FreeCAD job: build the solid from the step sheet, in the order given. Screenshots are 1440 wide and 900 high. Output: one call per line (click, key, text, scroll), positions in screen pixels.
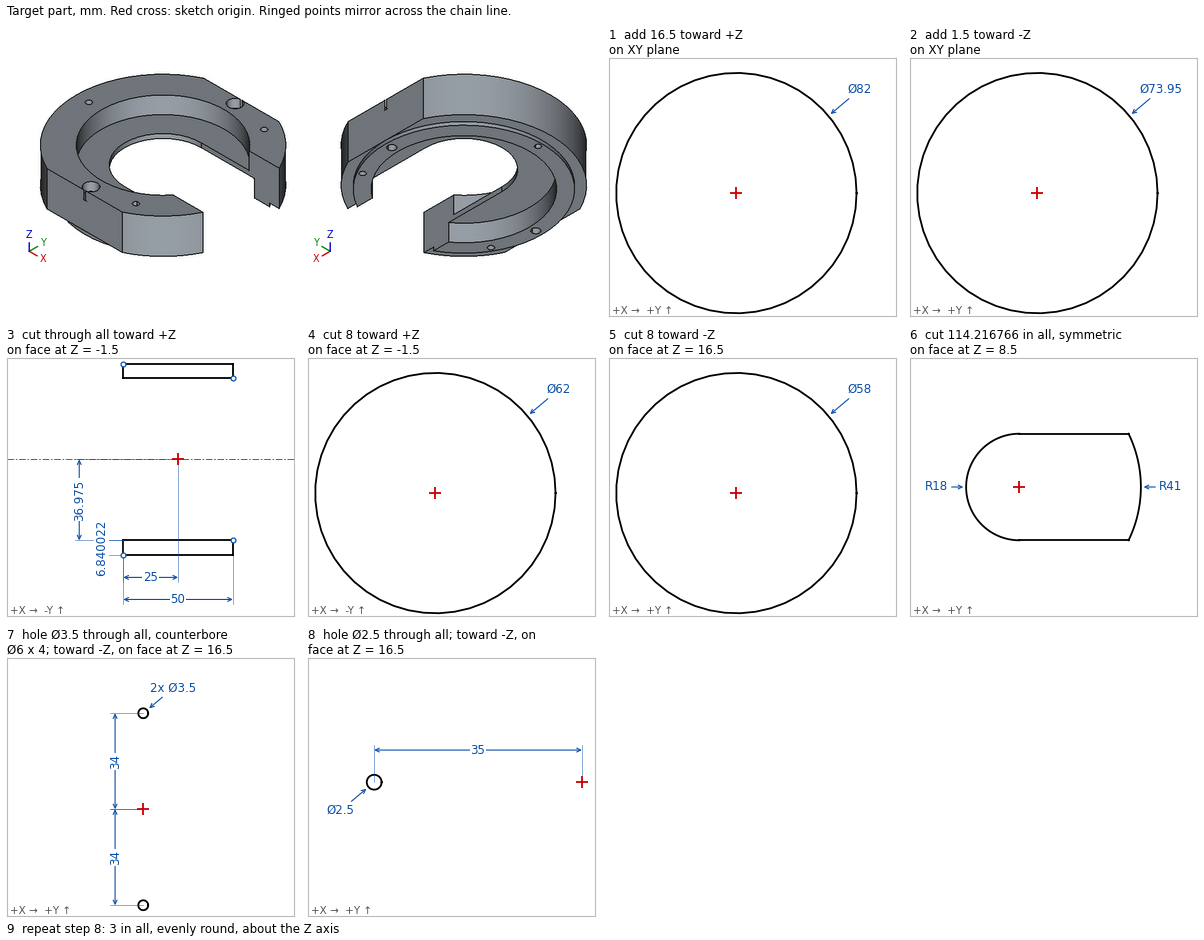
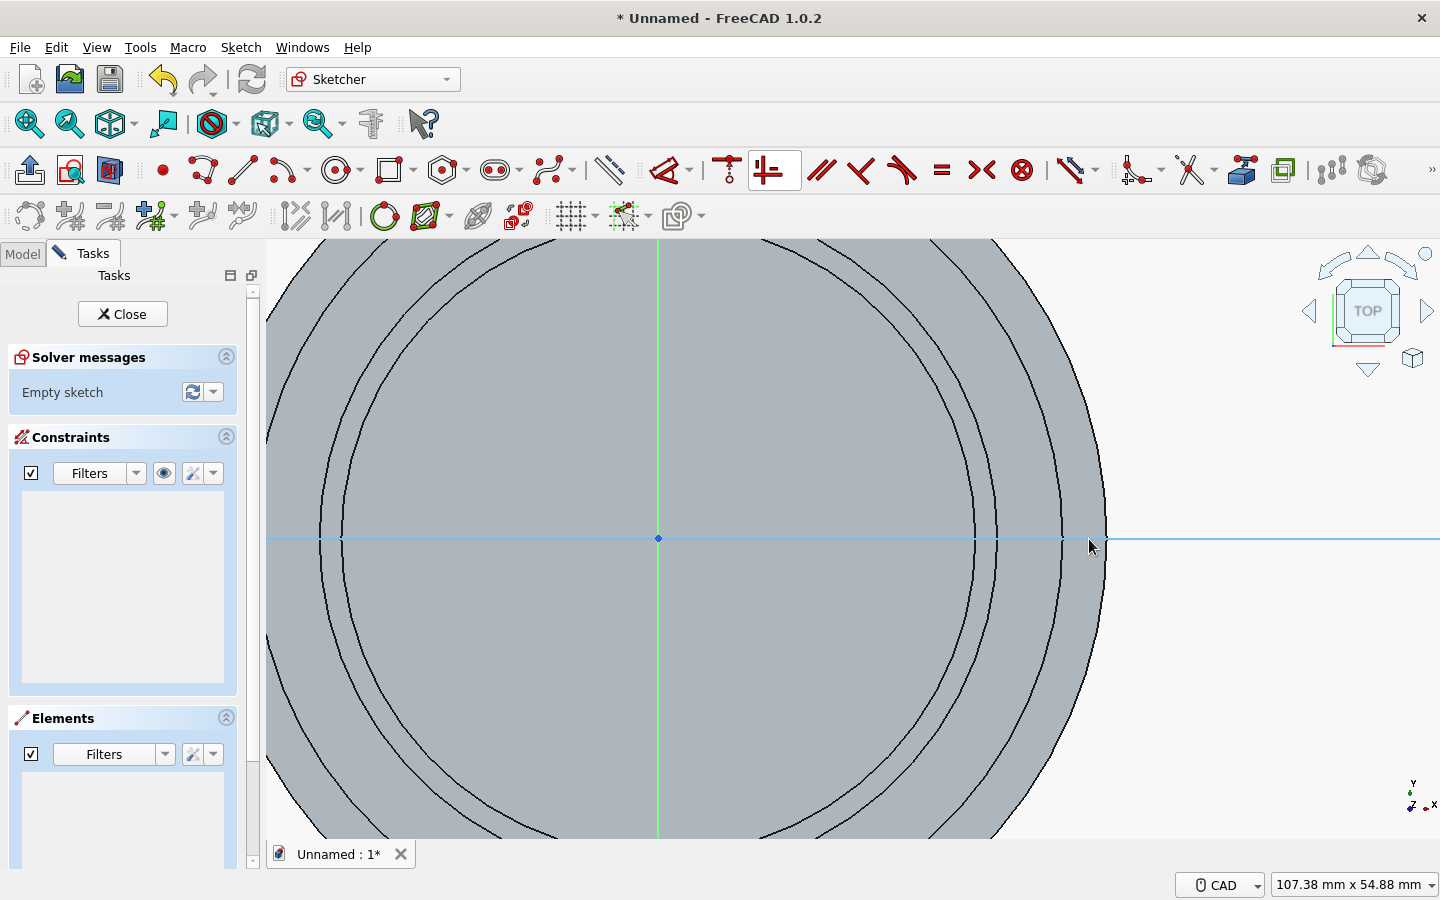
key(g)
key(l)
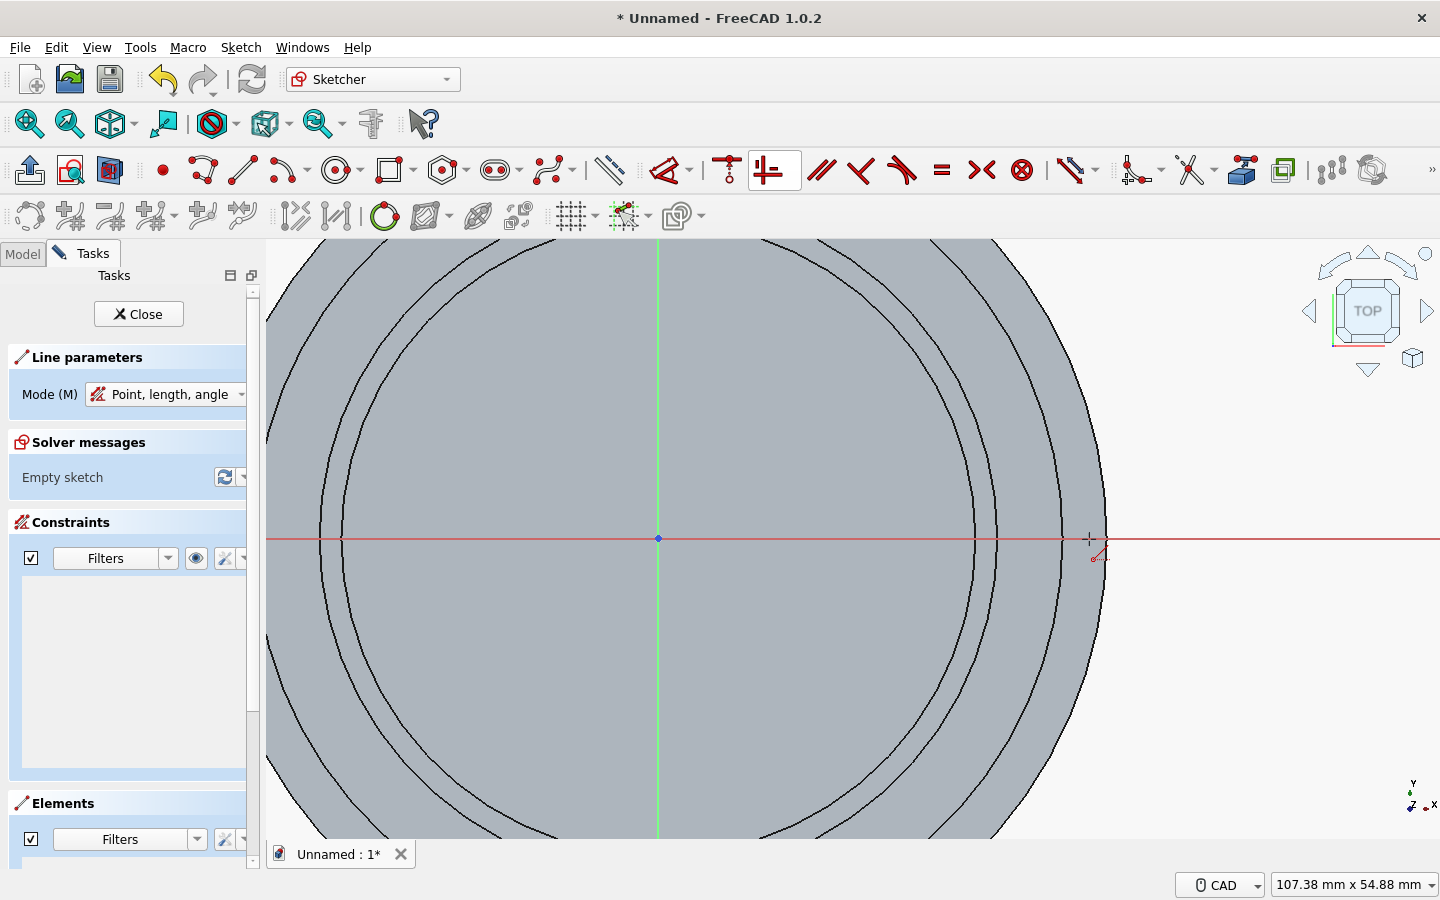
click(1061, 342)
click(658, 342)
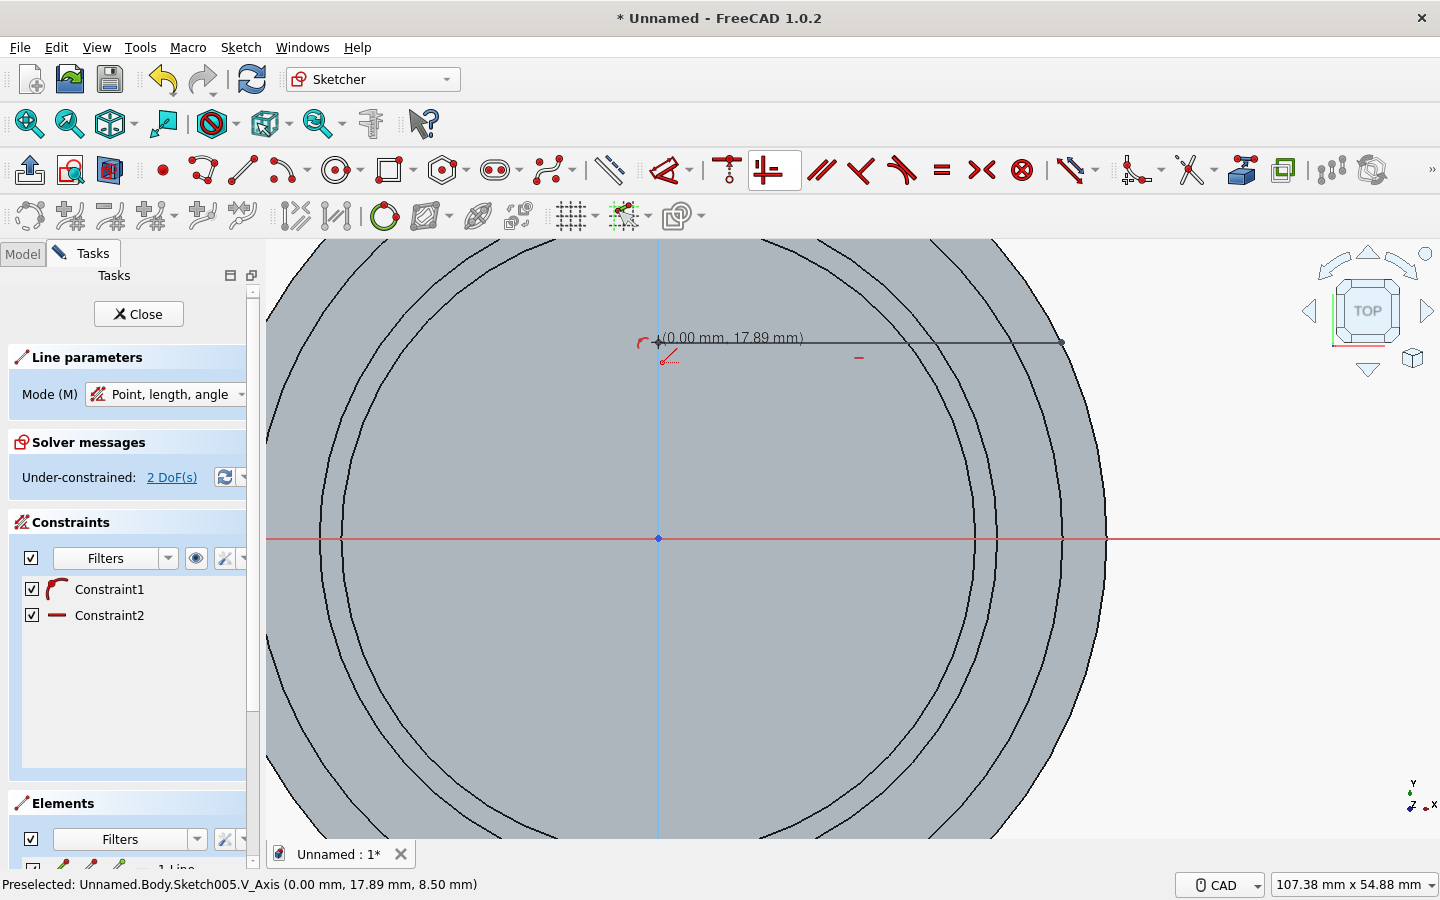
click(658, 735)
click(1061, 735)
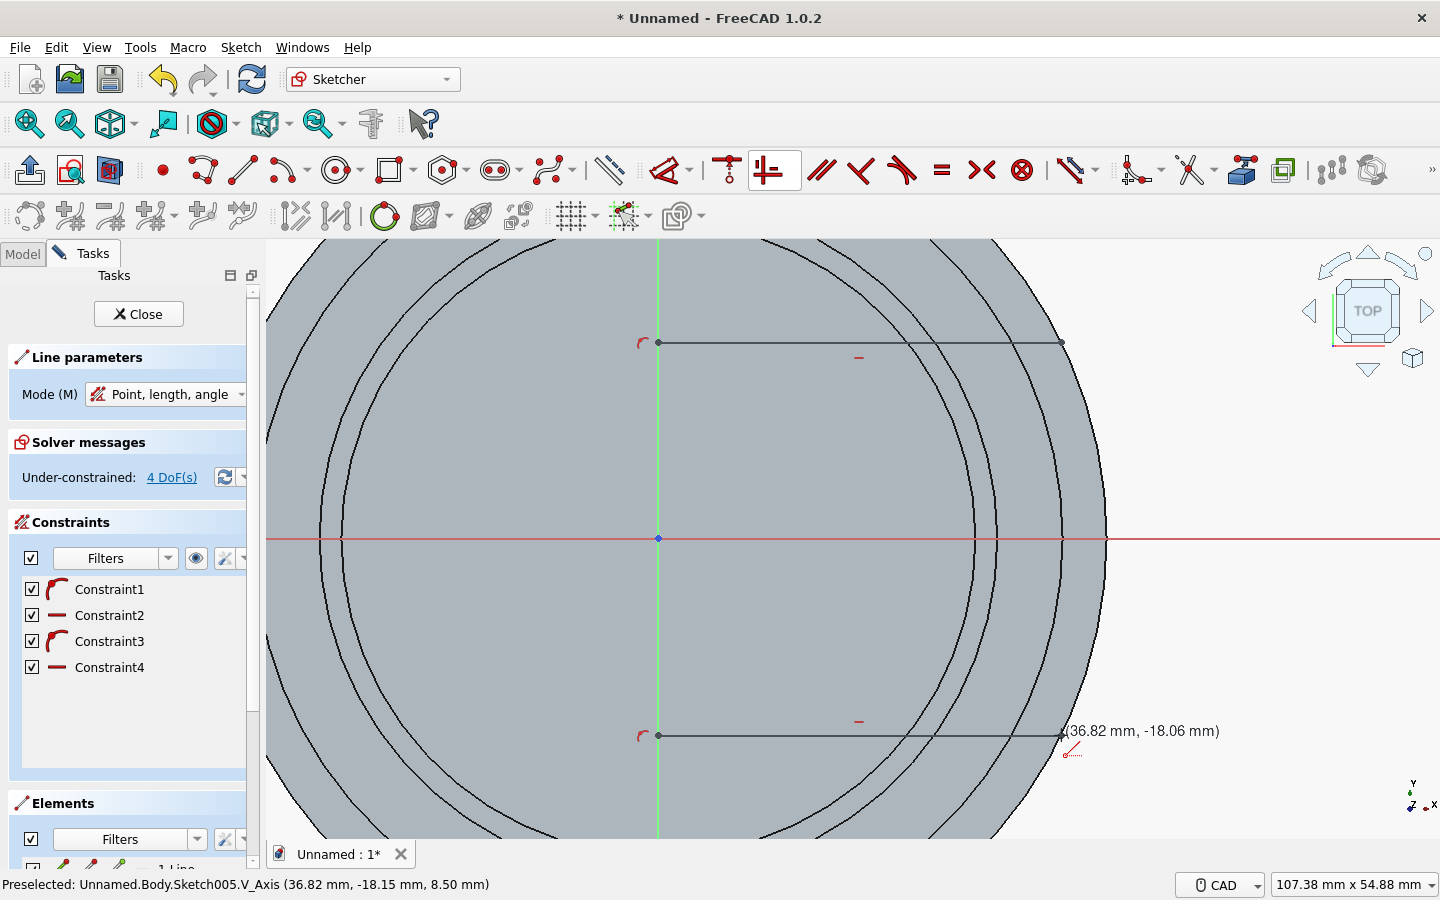
key(g)
key(3)
key(a)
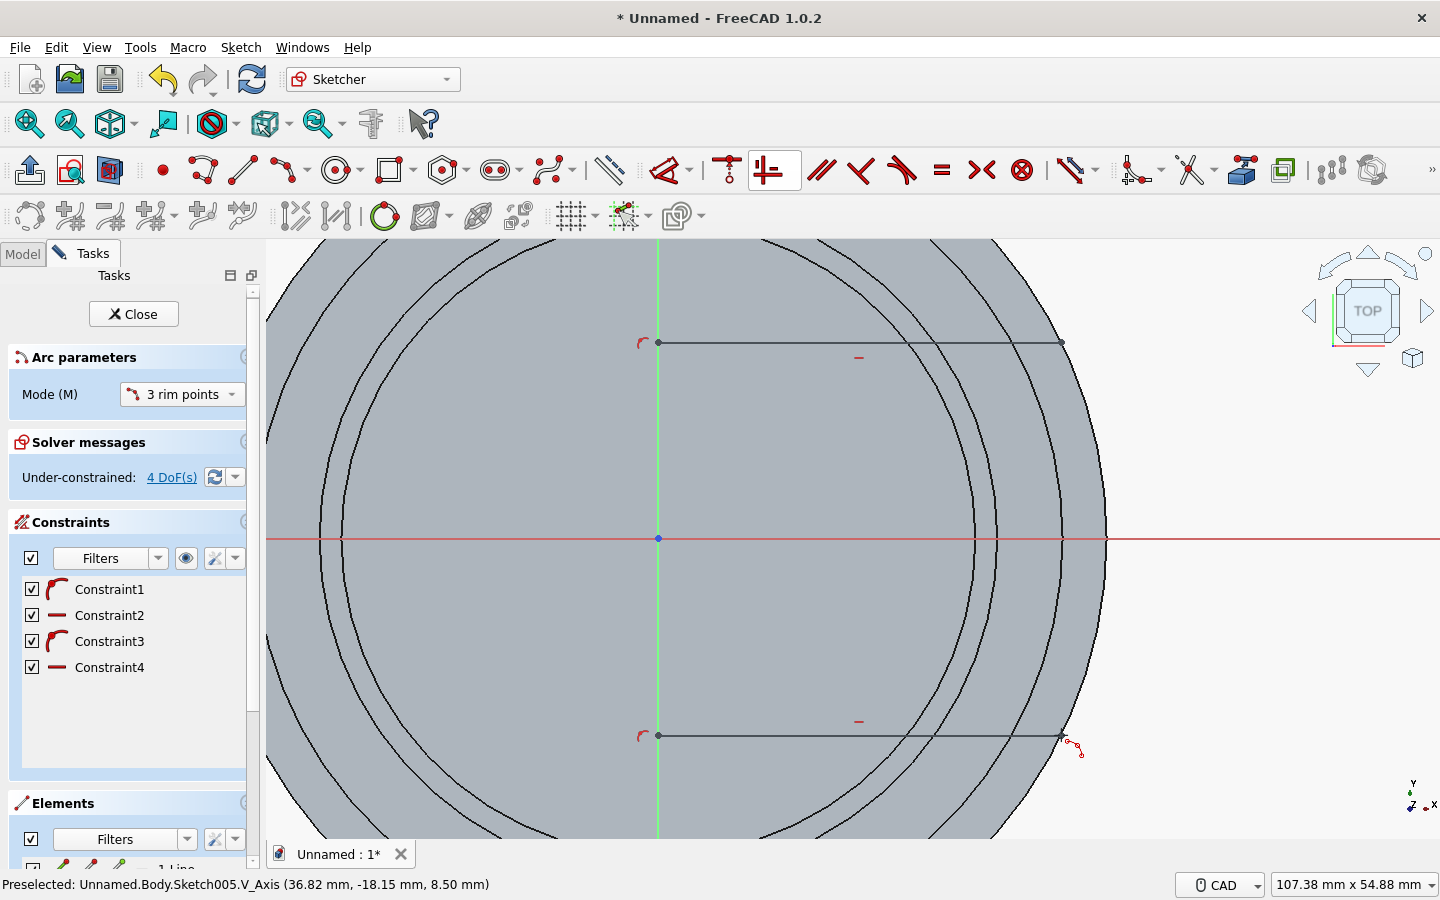
click(658, 343)
click(658, 736)
click(471, 478)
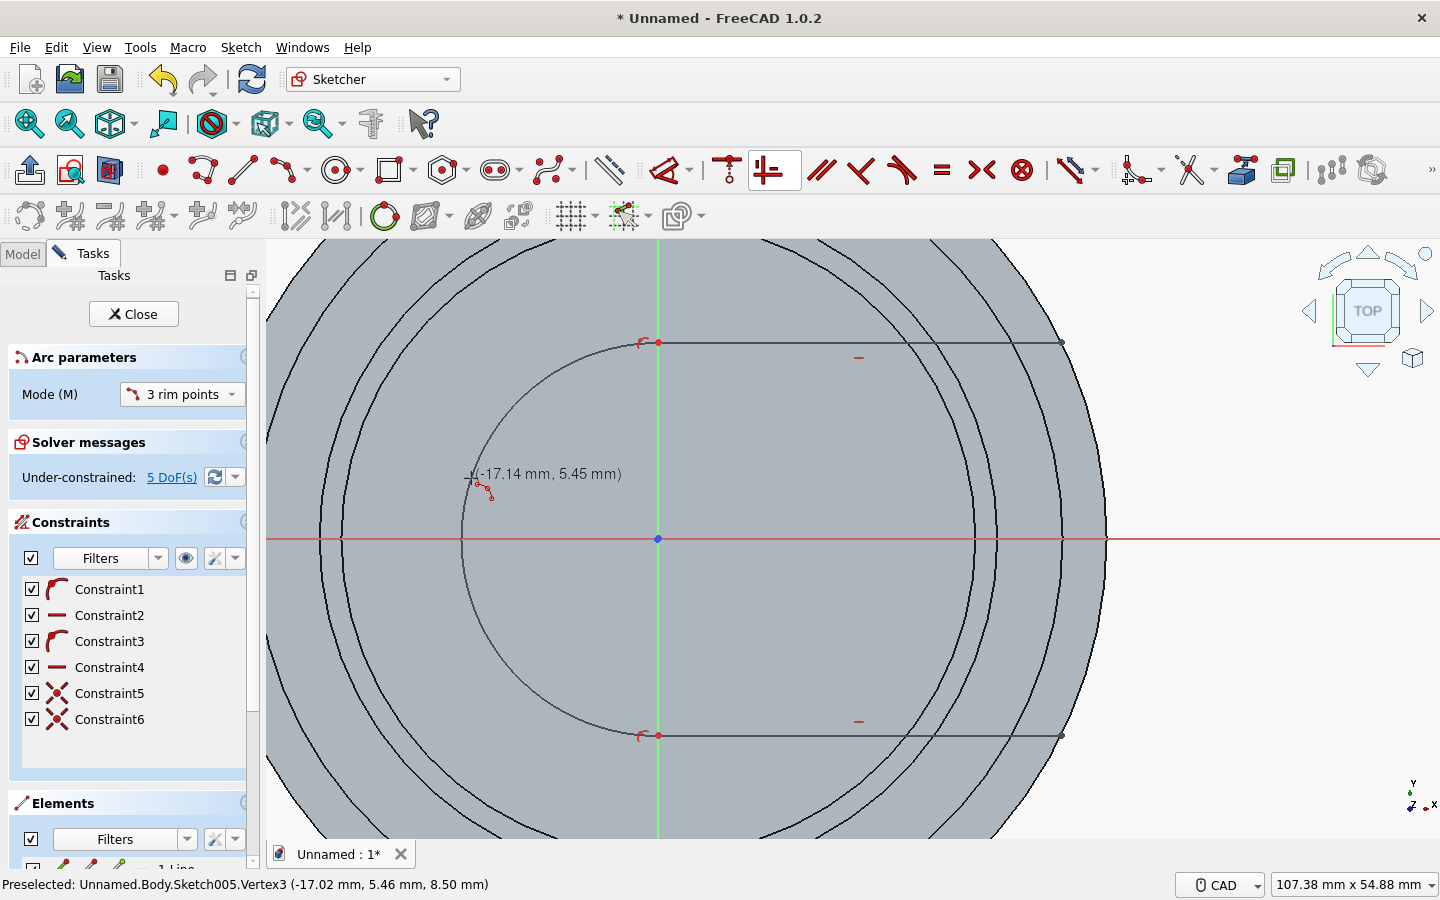
click(1061, 736)
click(1061, 343)
click(1105, 579)
key(Escape)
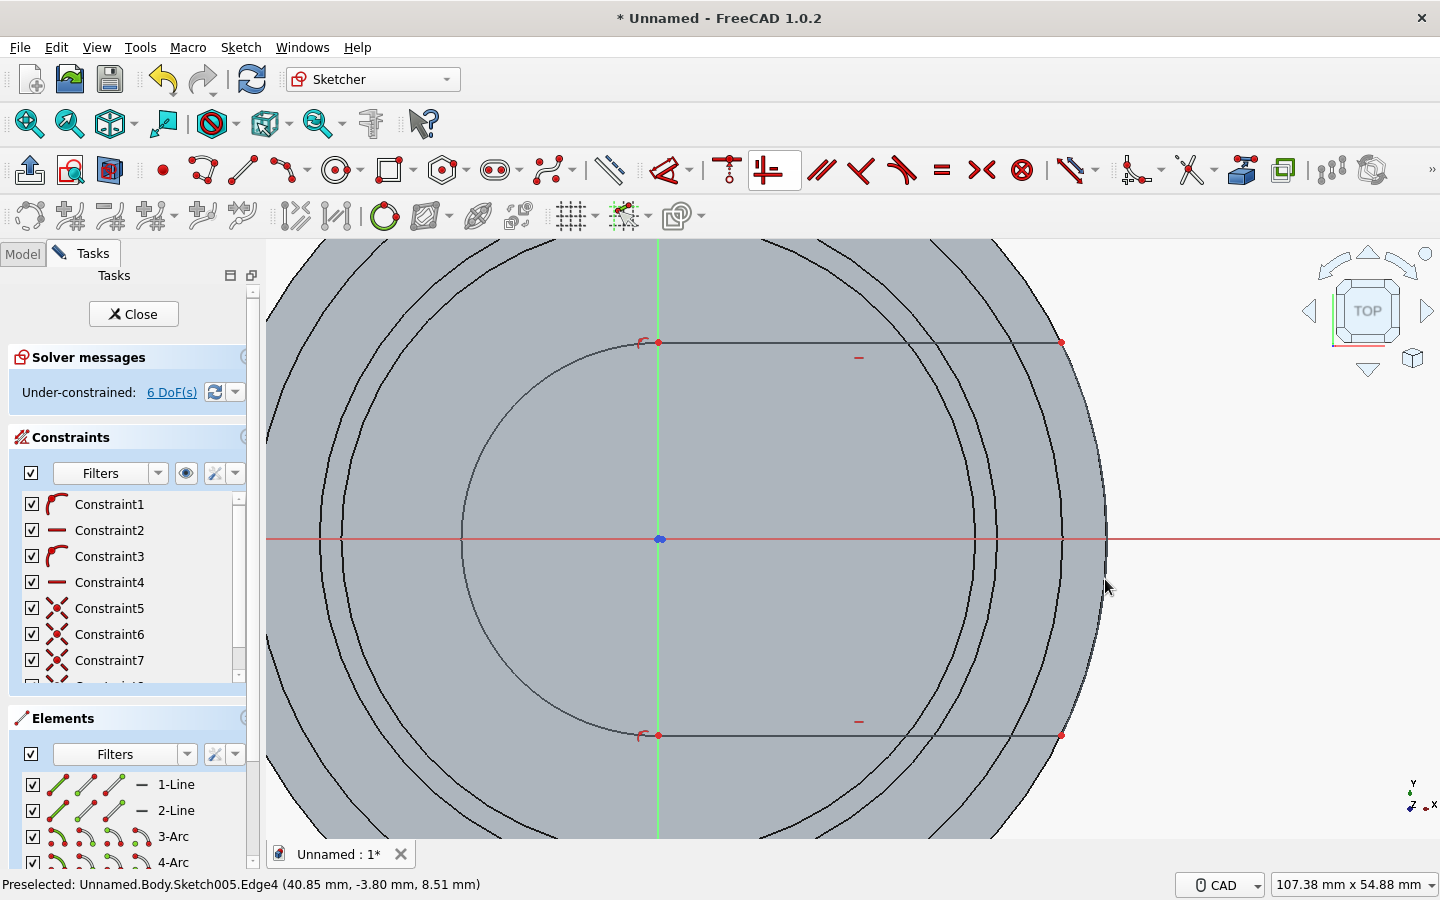
click(940, 343)